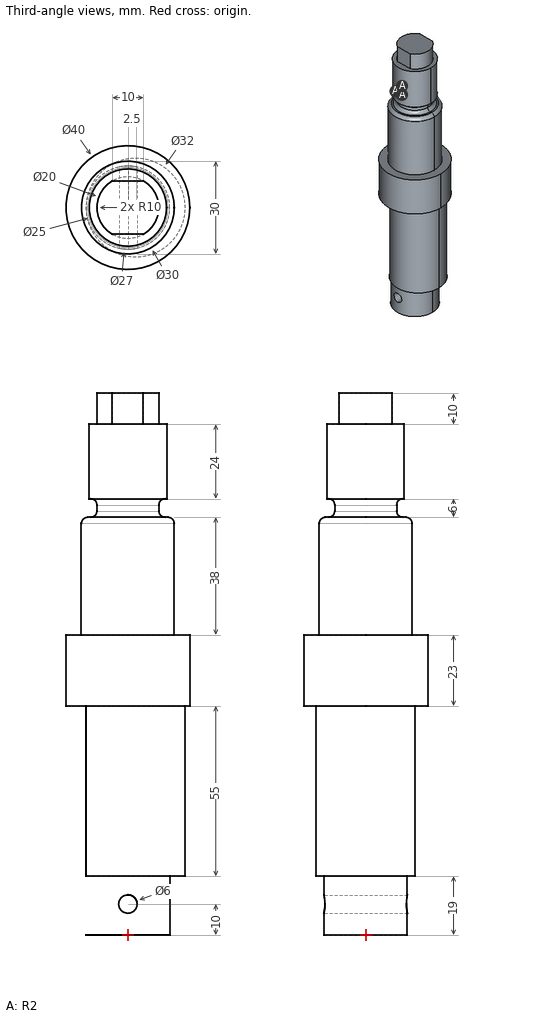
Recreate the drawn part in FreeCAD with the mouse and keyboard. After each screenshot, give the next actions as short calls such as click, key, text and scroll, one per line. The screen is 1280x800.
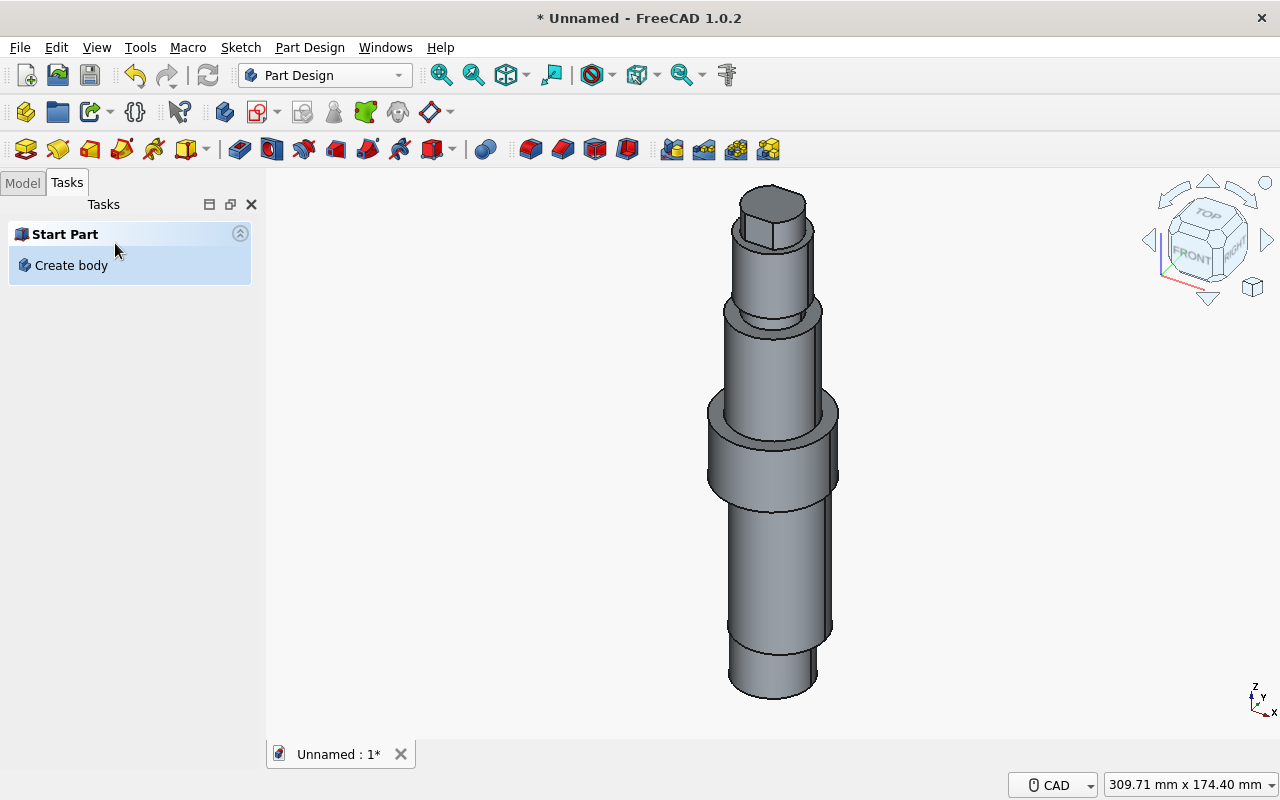
key(v)
key(f)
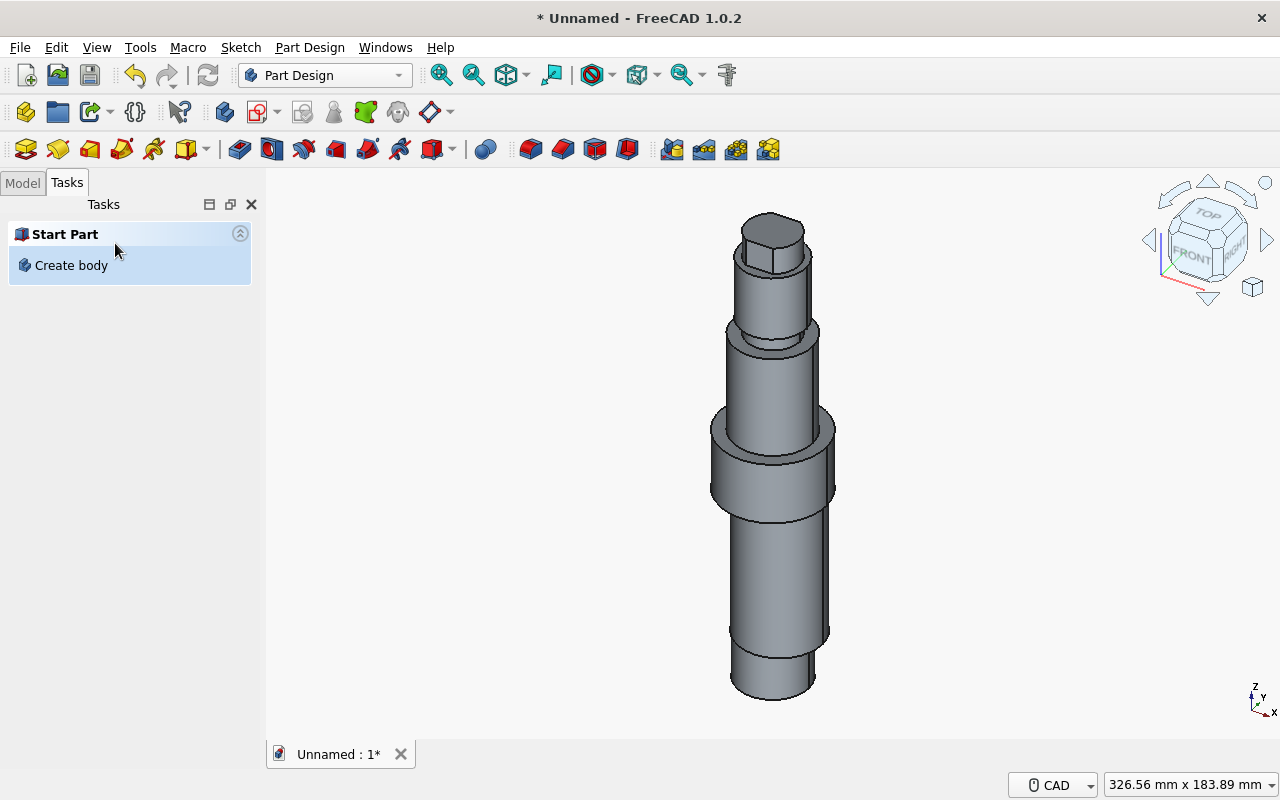
click(258, 112)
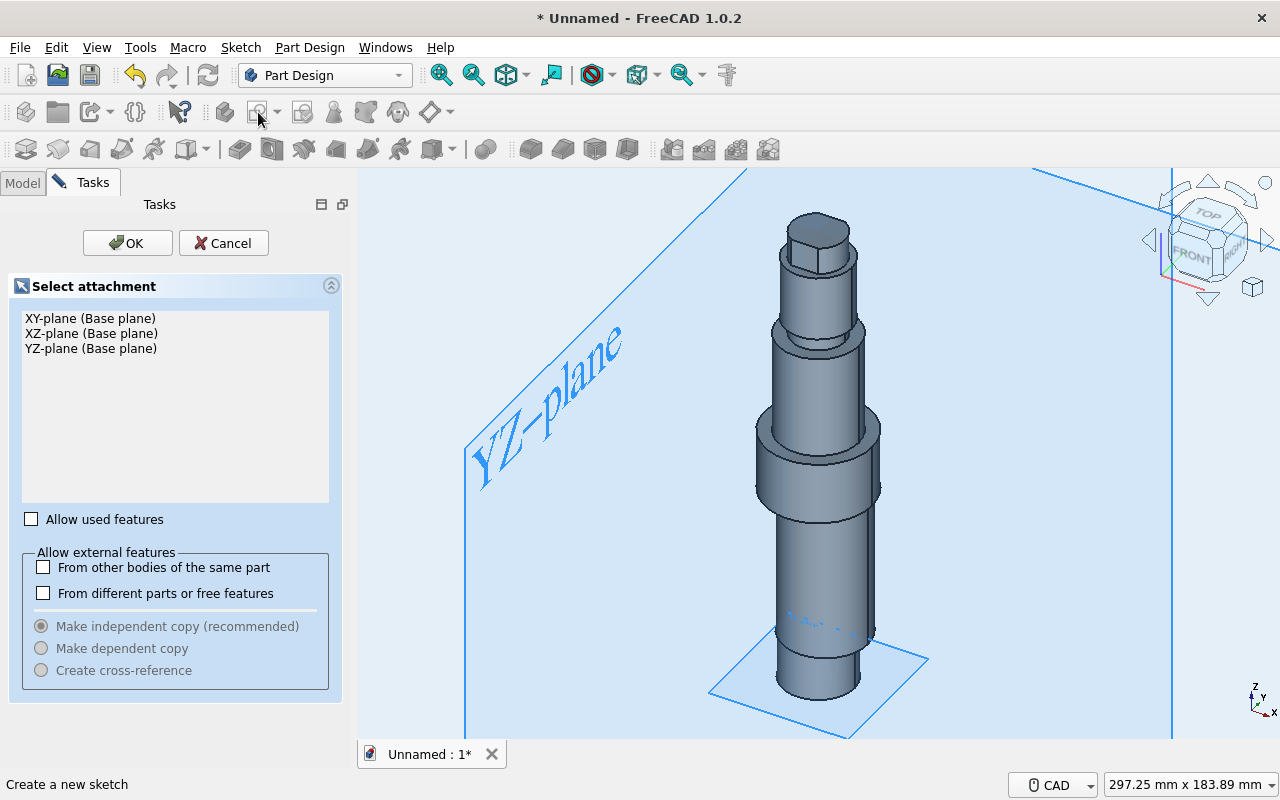
click(82, 334)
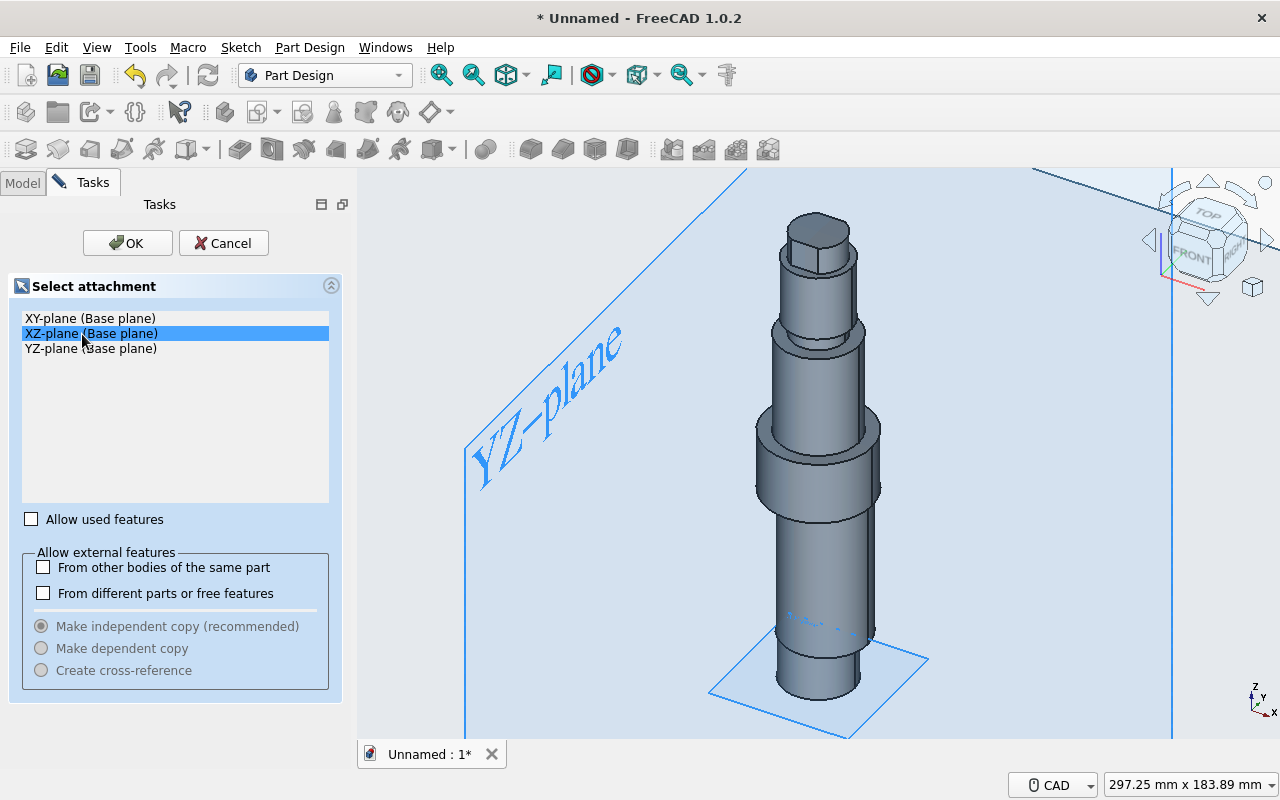
click(128, 243)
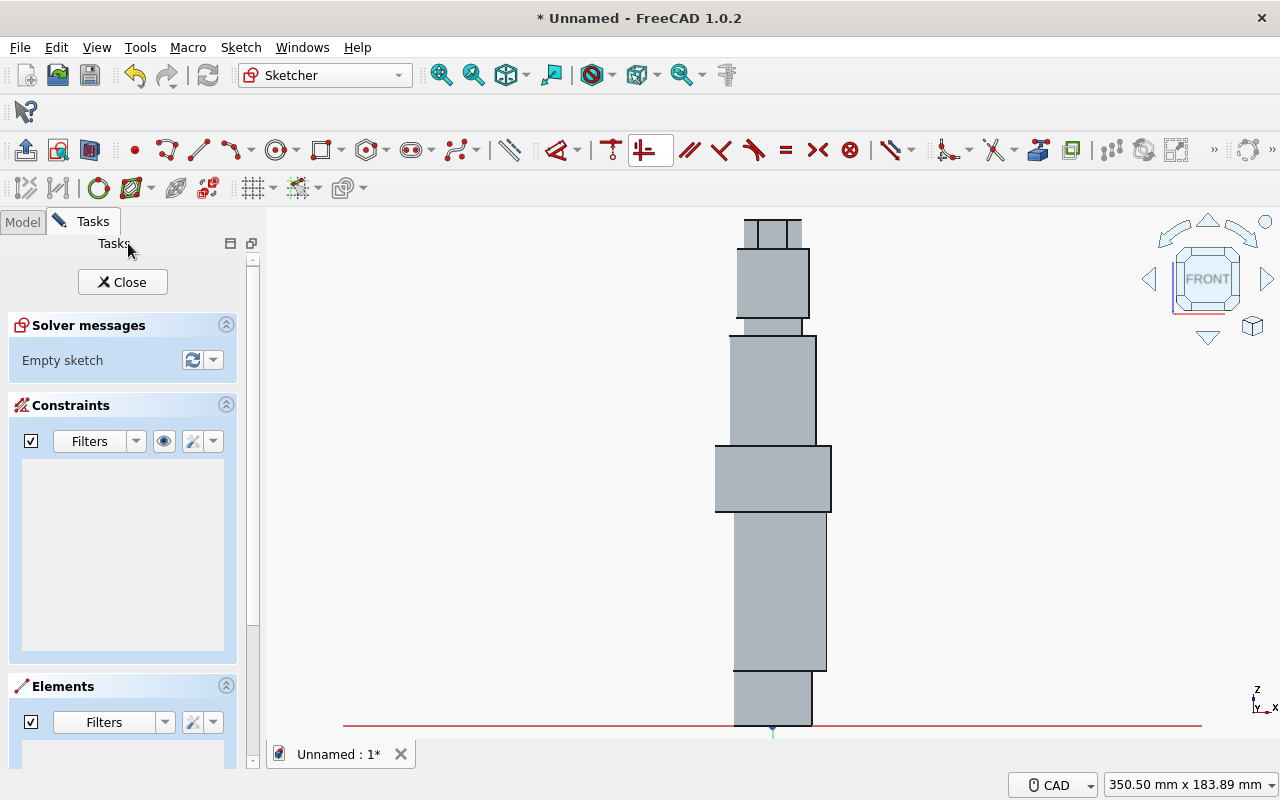
key(q)
key(s)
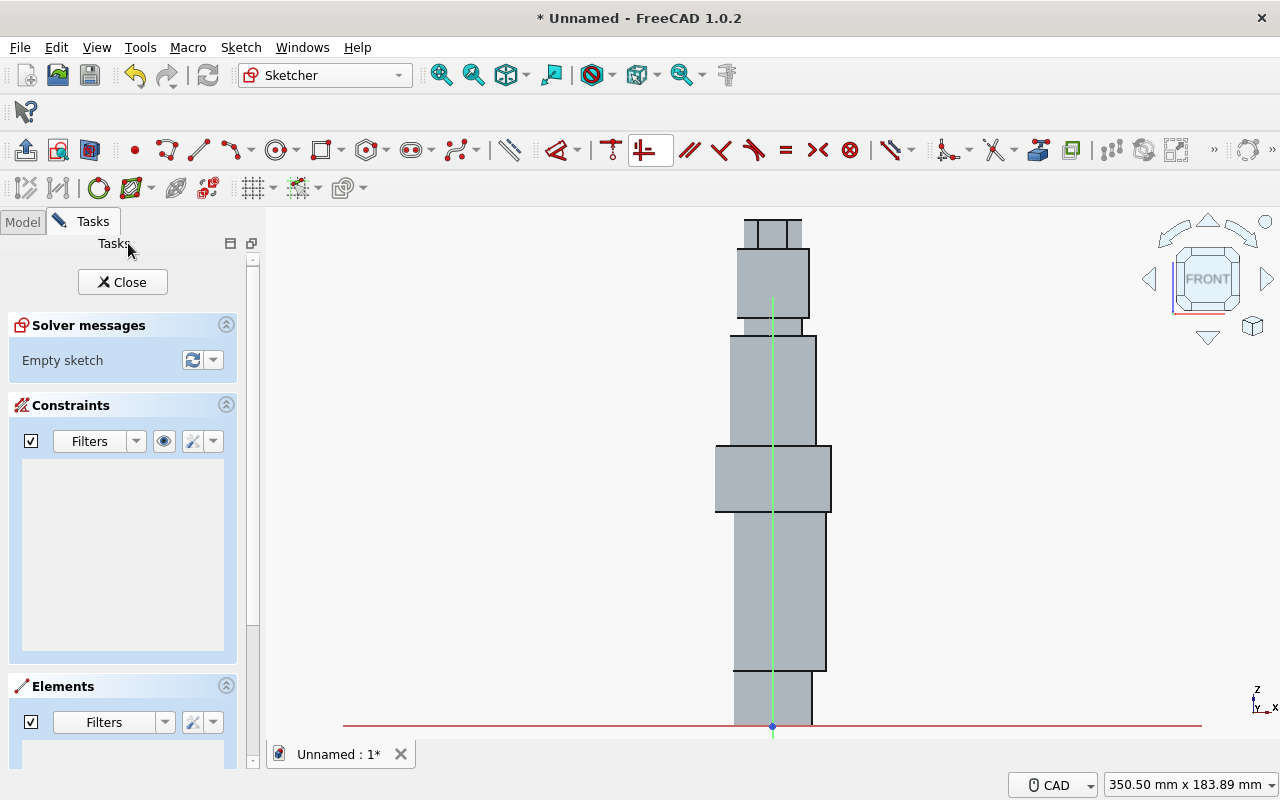
scroll(704, 473, down, 5)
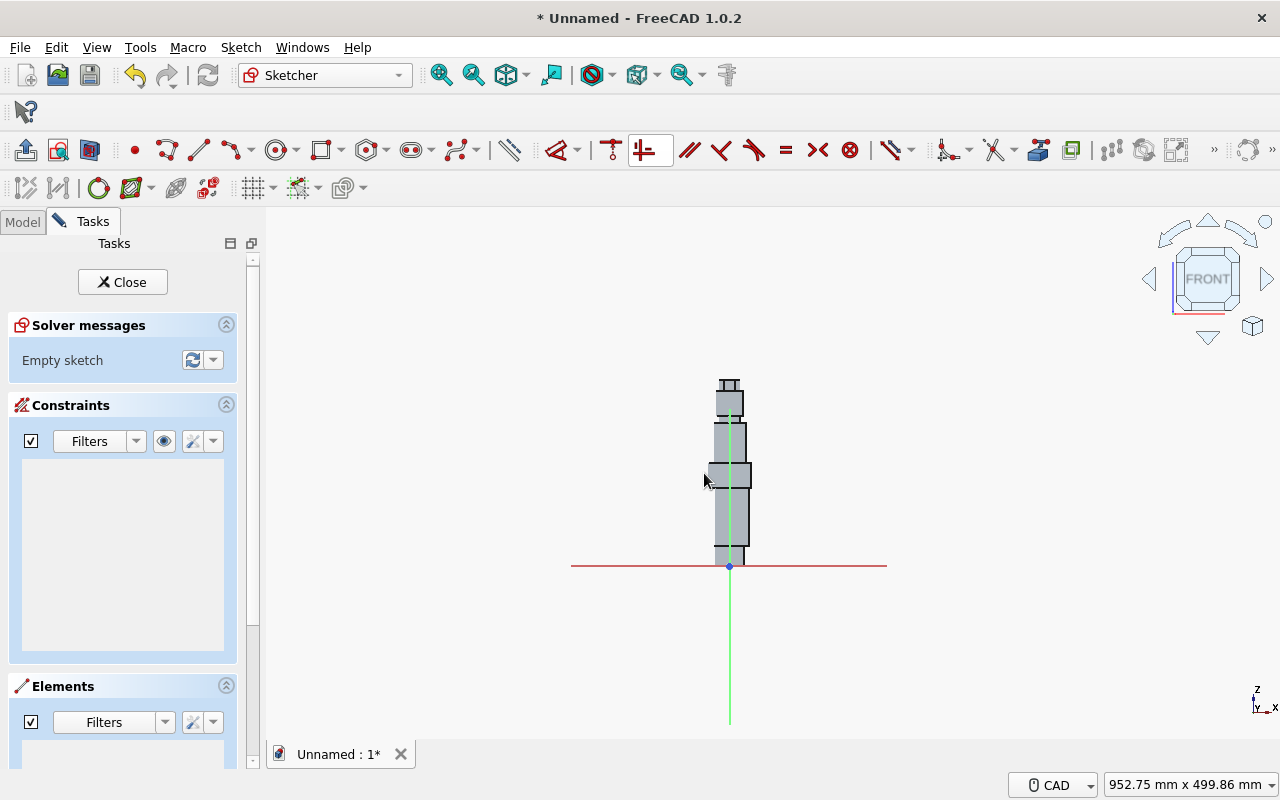
scroll(731, 564, up, 15)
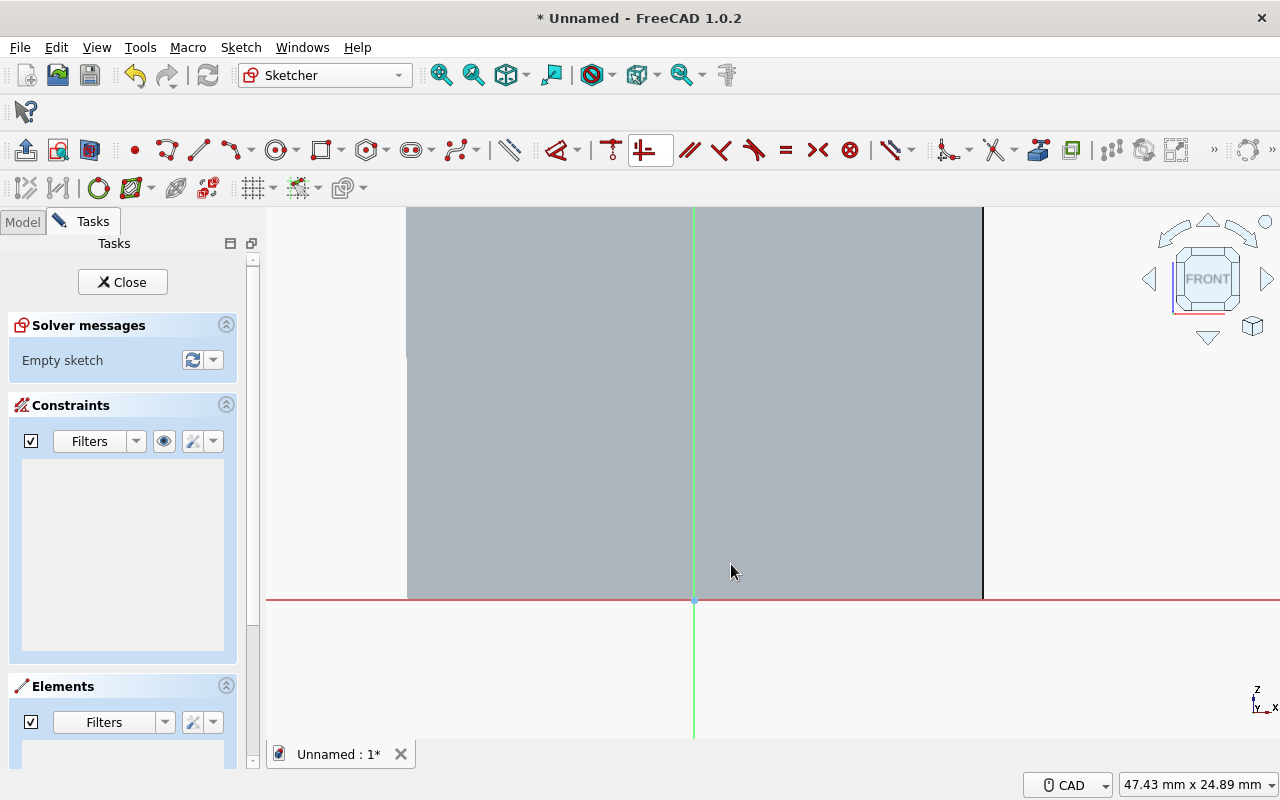
key(g)
key(c)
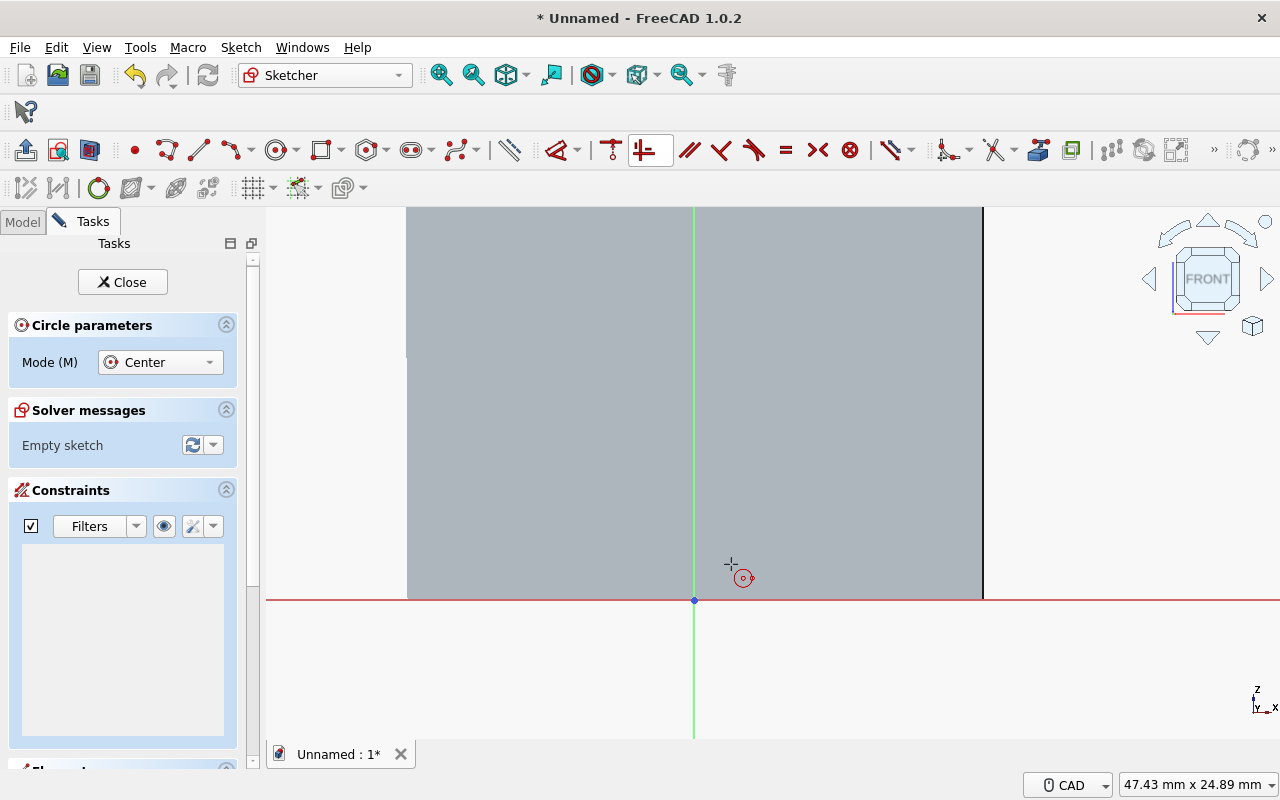
click(694, 386)
click(740, 341)
key(Escape)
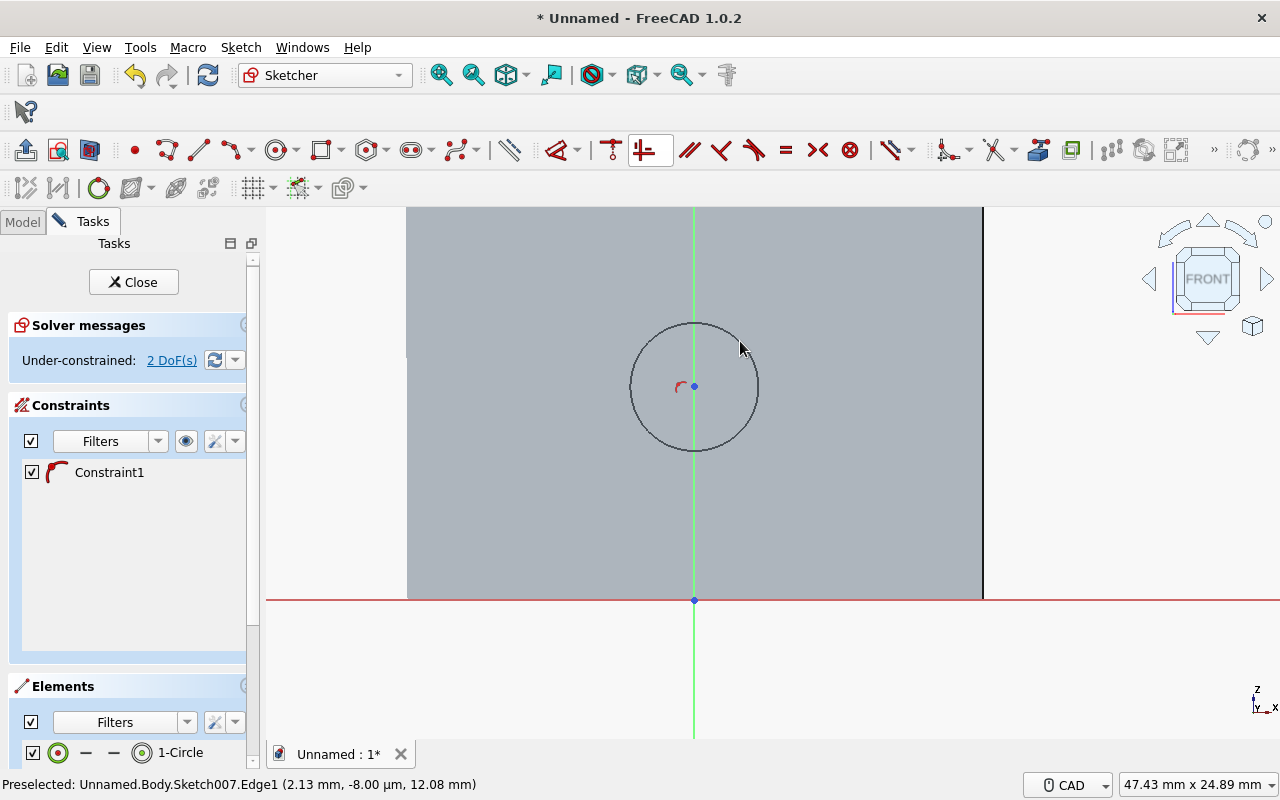
key(d)